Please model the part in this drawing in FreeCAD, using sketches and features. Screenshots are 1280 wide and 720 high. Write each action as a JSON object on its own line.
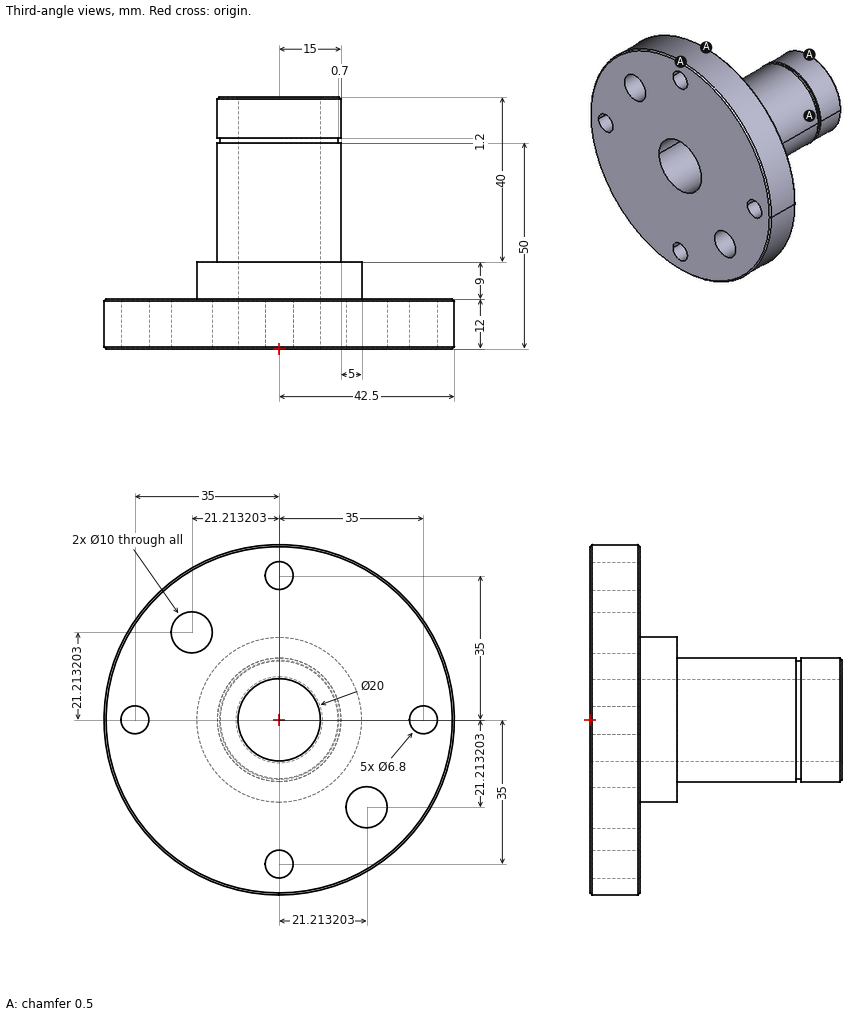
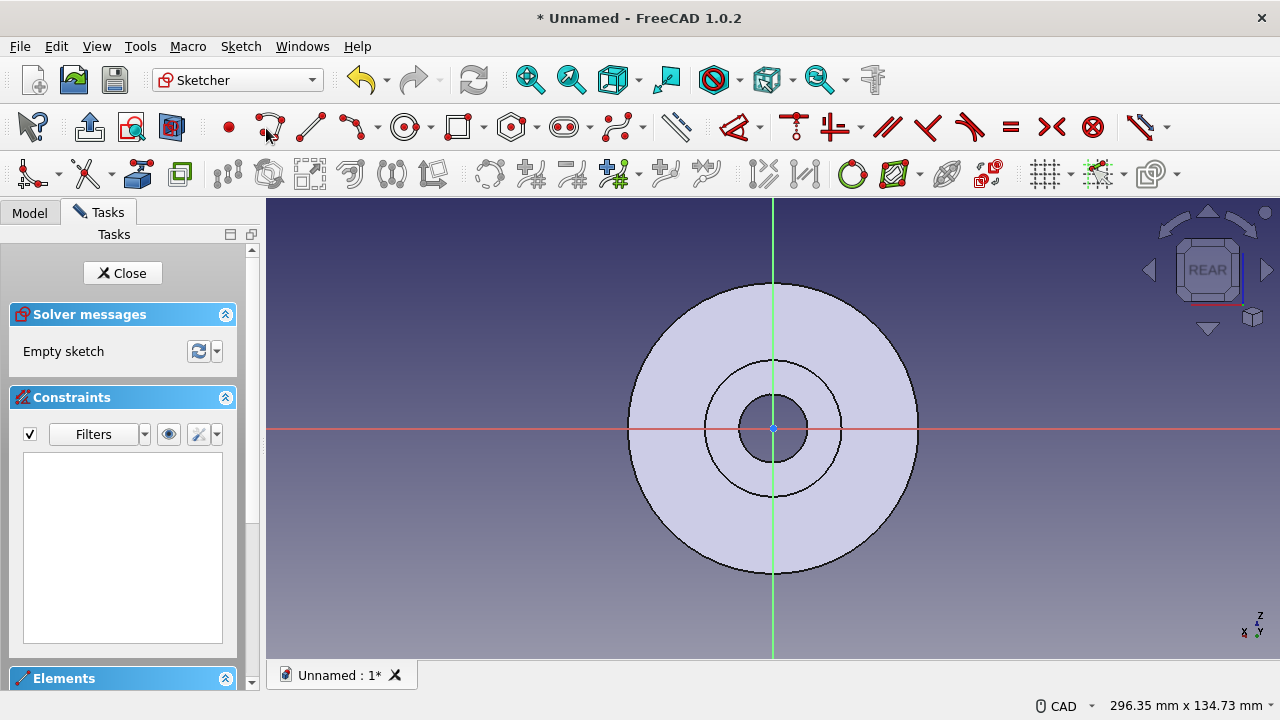
{"action": "key", "text": "g c"}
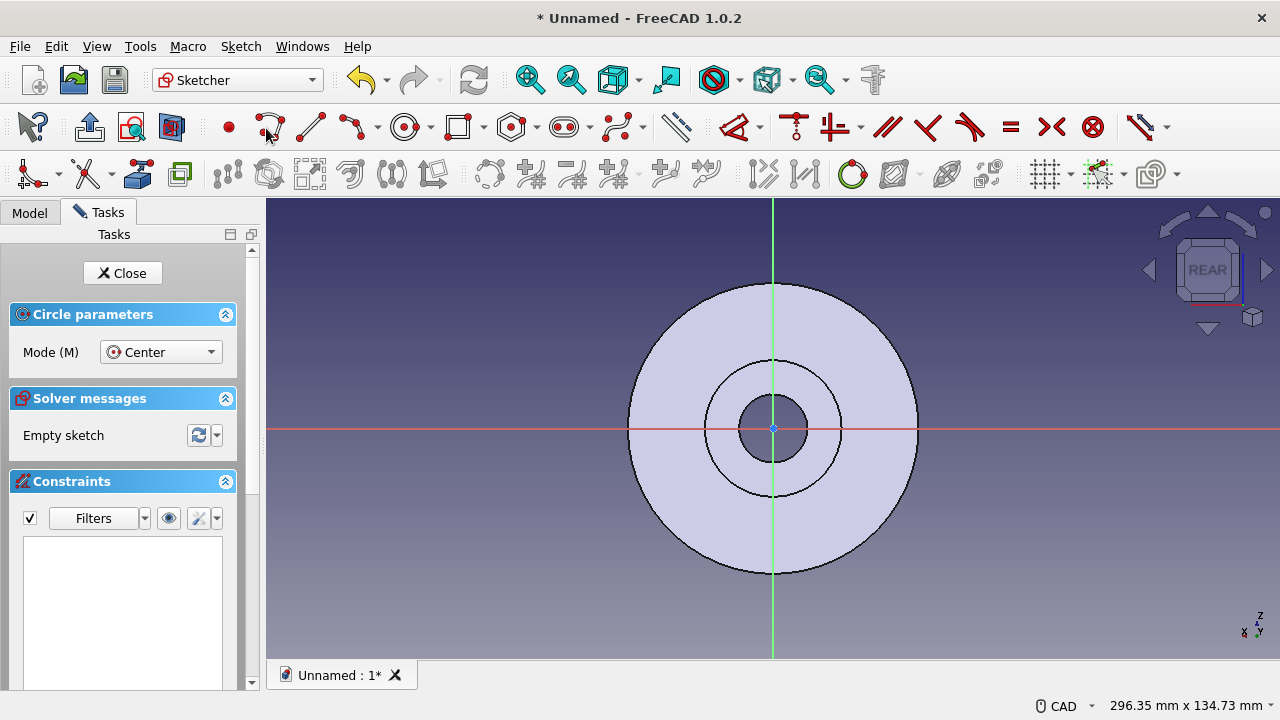
{"action": "scroll", "coordinate": [653, 429], "scroll_direction": "up", "scroll_amount": 4}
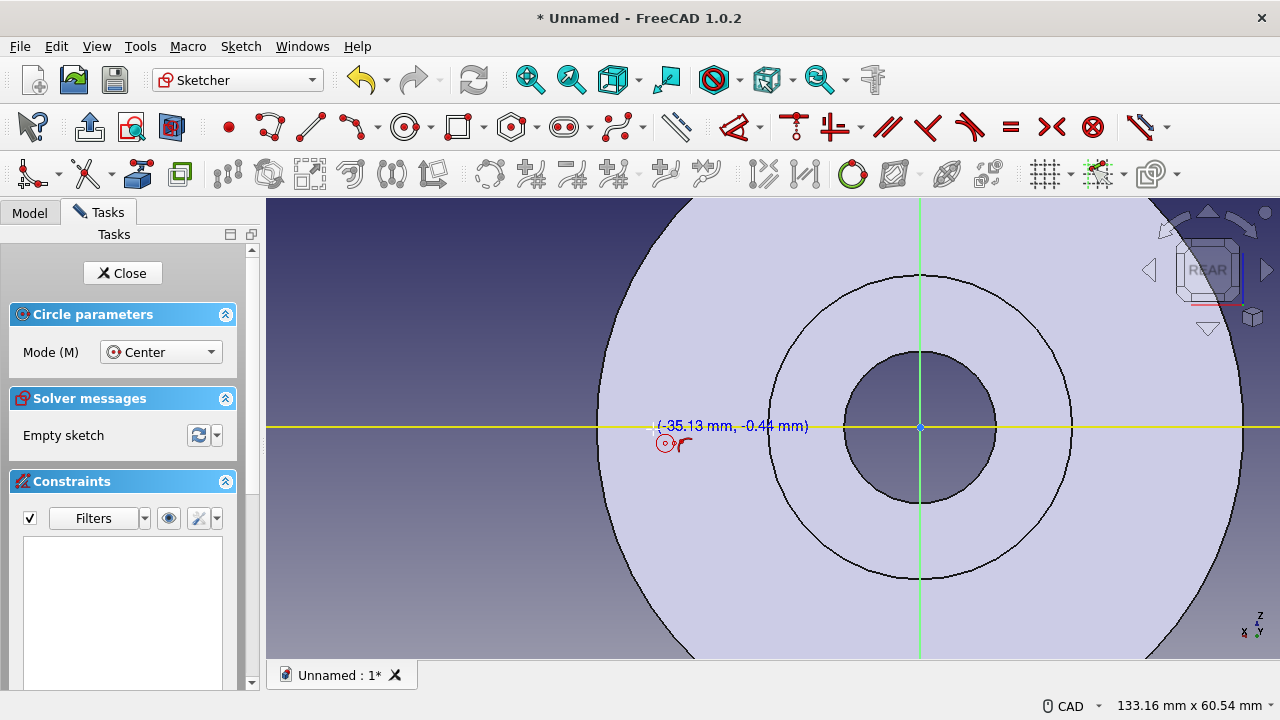
{"action": "left_click", "coordinate": [654, 427]}
{"action": "left_click", "coordinate": [672, 409]}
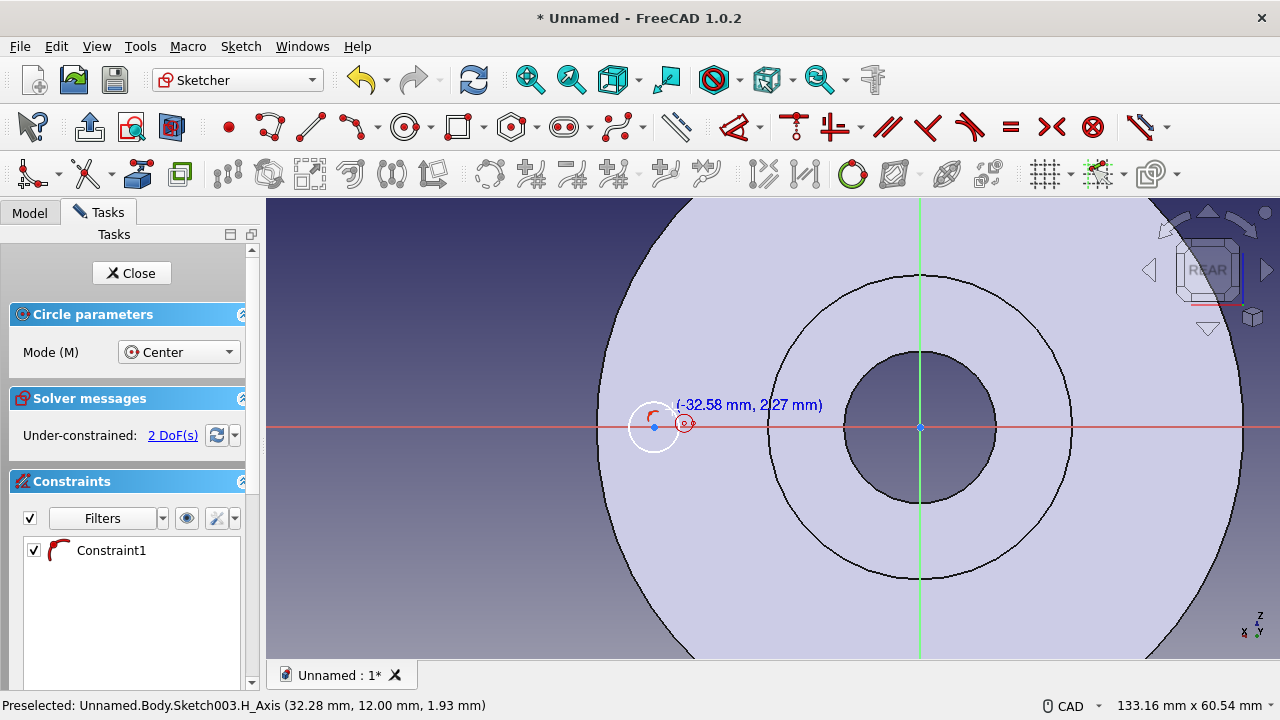
{"action": "scroll", "coordinate": [529, 430], "scroll_direction": "down", "scroll_amount": 4}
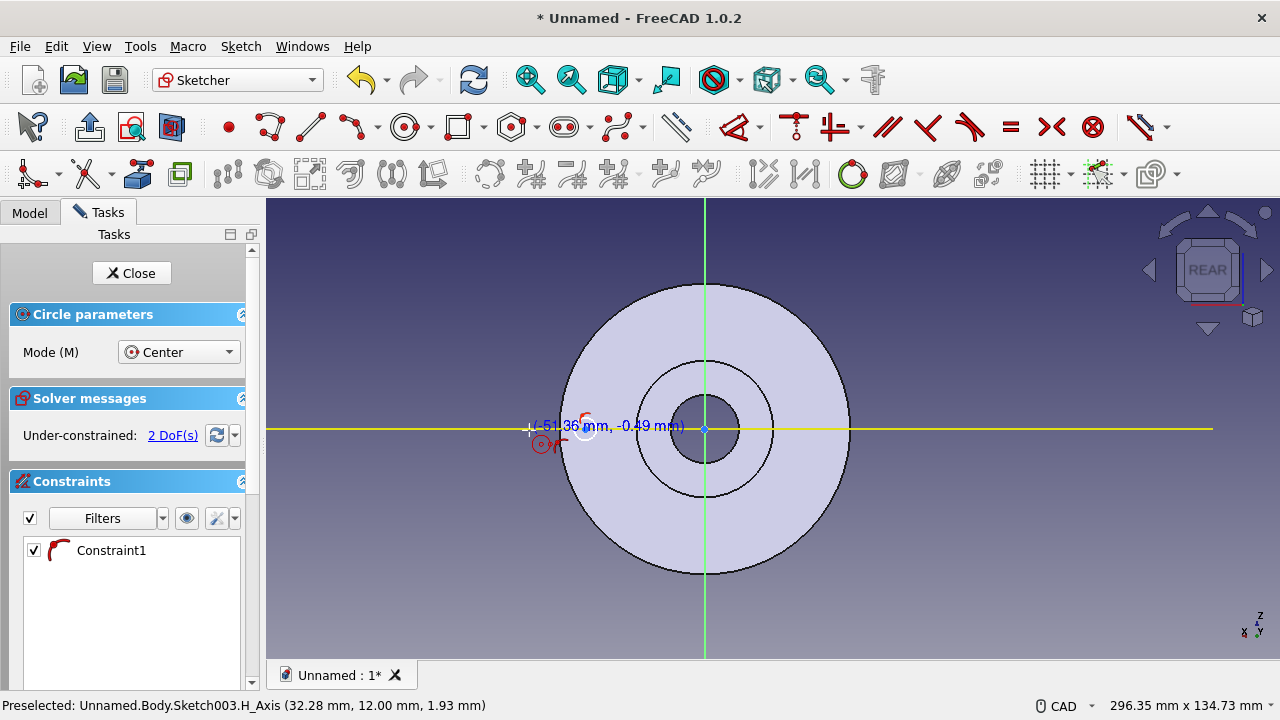
{"action": "scroll", "coordinate": [705, 309], "scroll_direction": "up", "scroll_amount": 4}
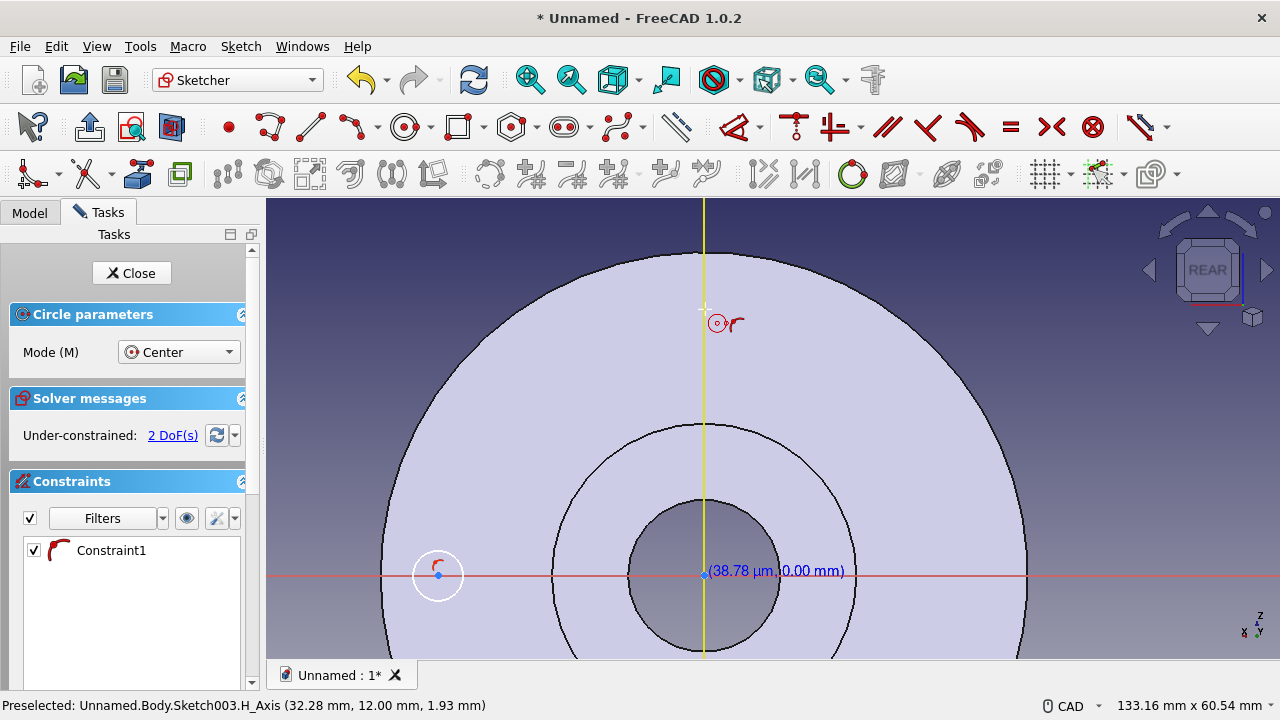
{"action": "left_click", "coordinate": [704, 309]}
{"action": "left_click", "coordinate": [722, 291]}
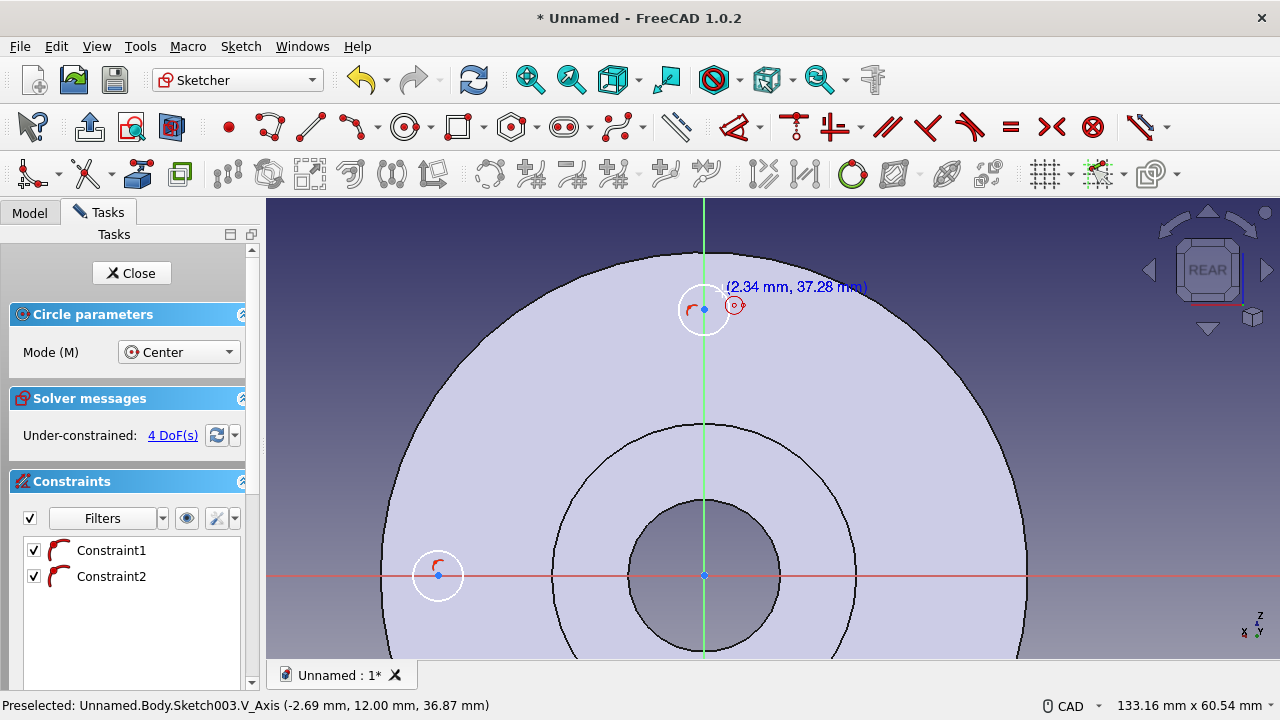
{"action": "left_click", "coordinate": [971, 576]}
{"action": "left_click", "coordinate": [989, 558]}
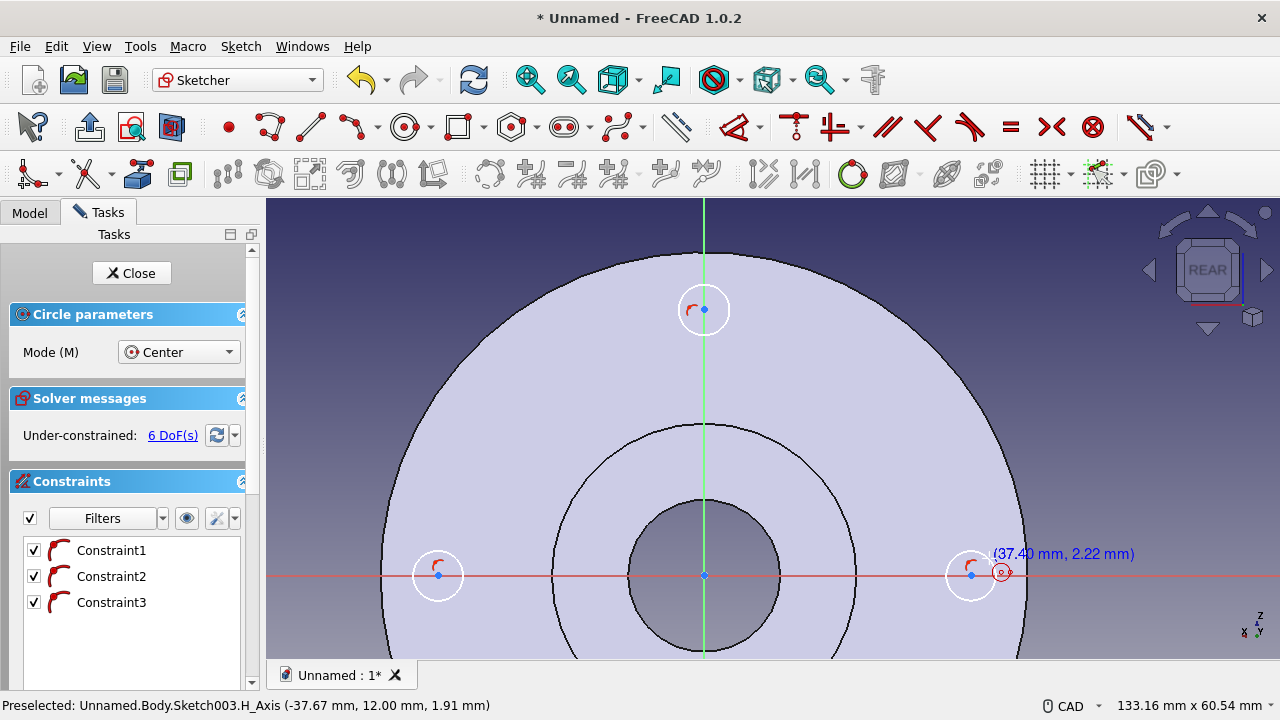
{"action": "scroll", "coordinate": [705, 308], "scroll_direction": "down", "scroll_amount": 4}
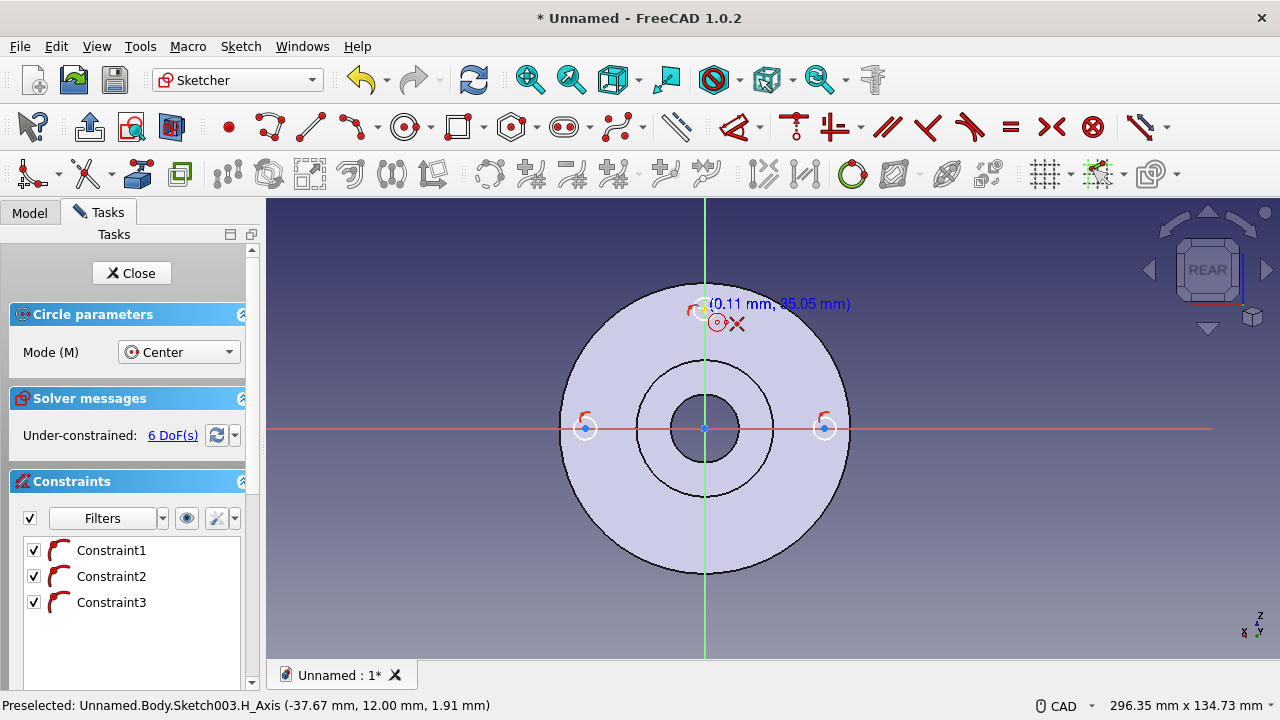
{"action": "scroll", "coordinate": [705, 548], "scroll_direction": "up", "scroll_amount": 4}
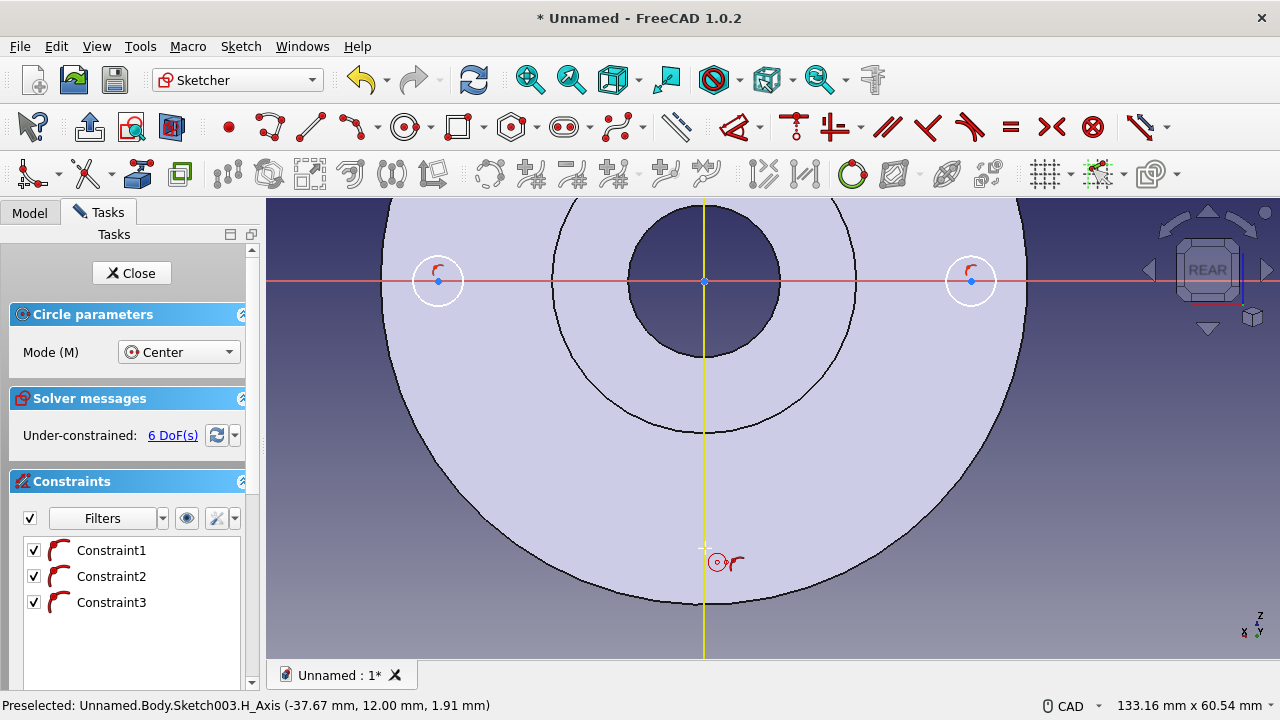
{"action": "left_click", "coordinate": [704, 548]}
{"action": "left_click", "coordinate": [722, 529]}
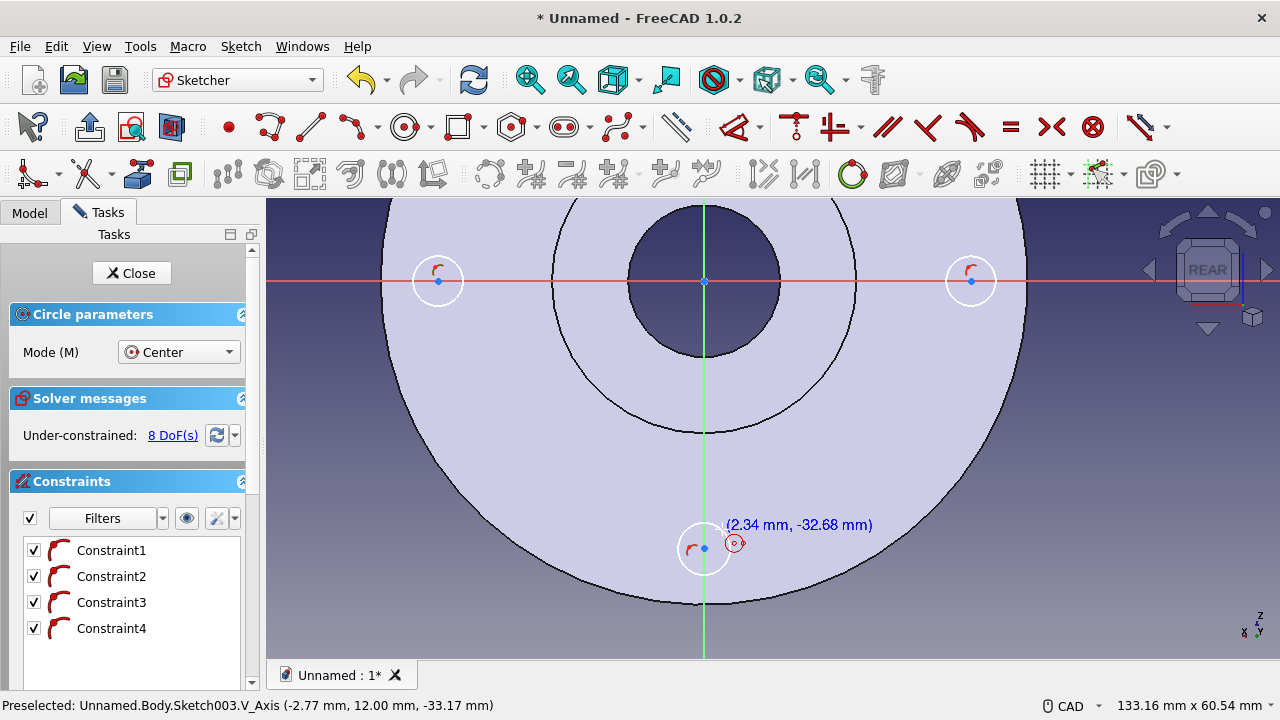
{"action": "left_click", "coordinate": [704, 281]}
{"action": "left_click", "coordinate": [722, 263]}
{"action": "key", "text": "Escape"}